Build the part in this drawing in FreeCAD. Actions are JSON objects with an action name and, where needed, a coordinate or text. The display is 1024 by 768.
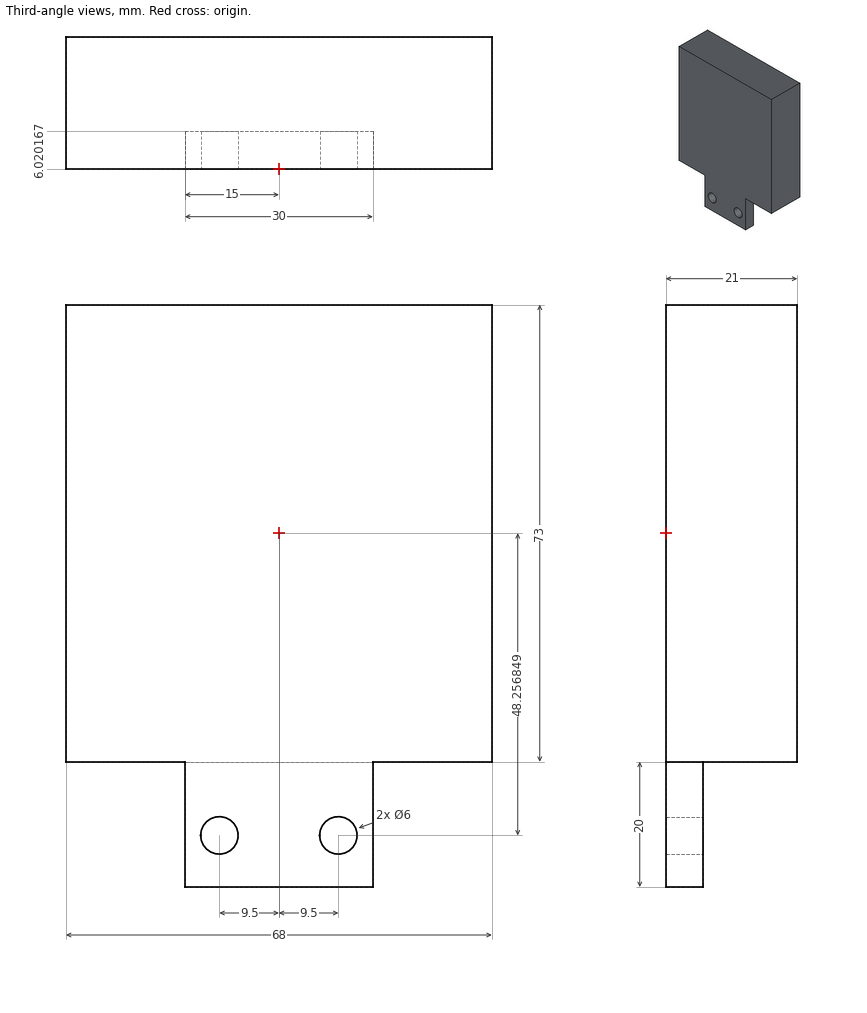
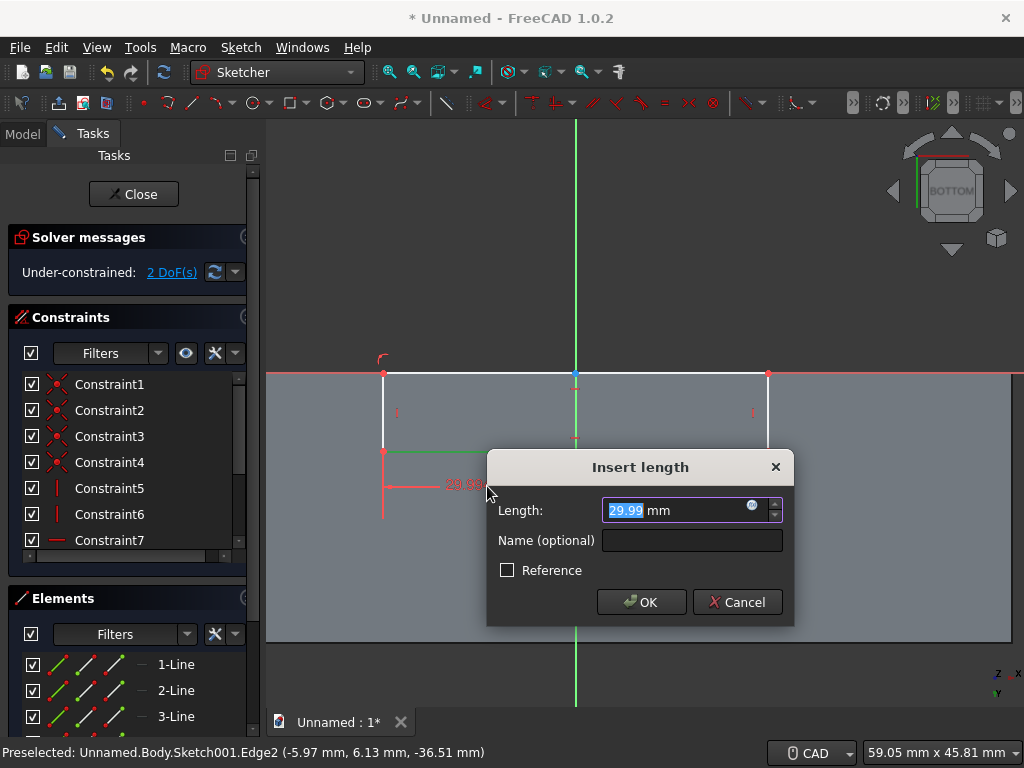
{"action": "type", "text": "30"}
{"action": "key", "text": "Return"}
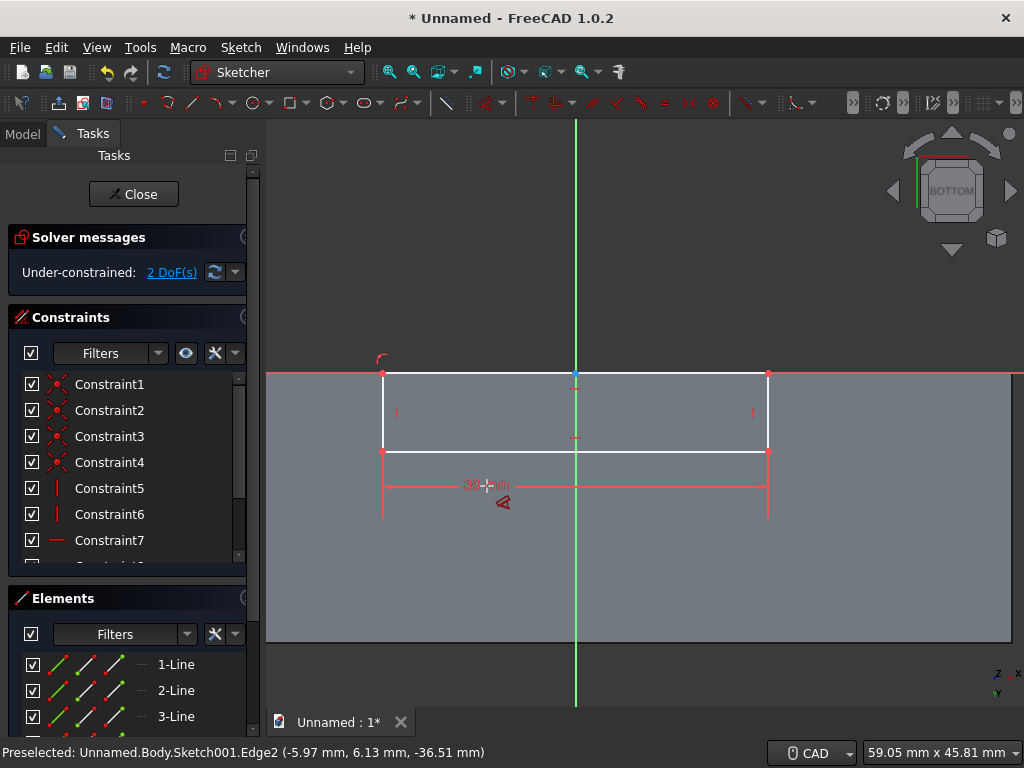
{"action": "left_click", "coordinate": [383, 373]}
{"action": "left_click", "coordinate": [479, 339]}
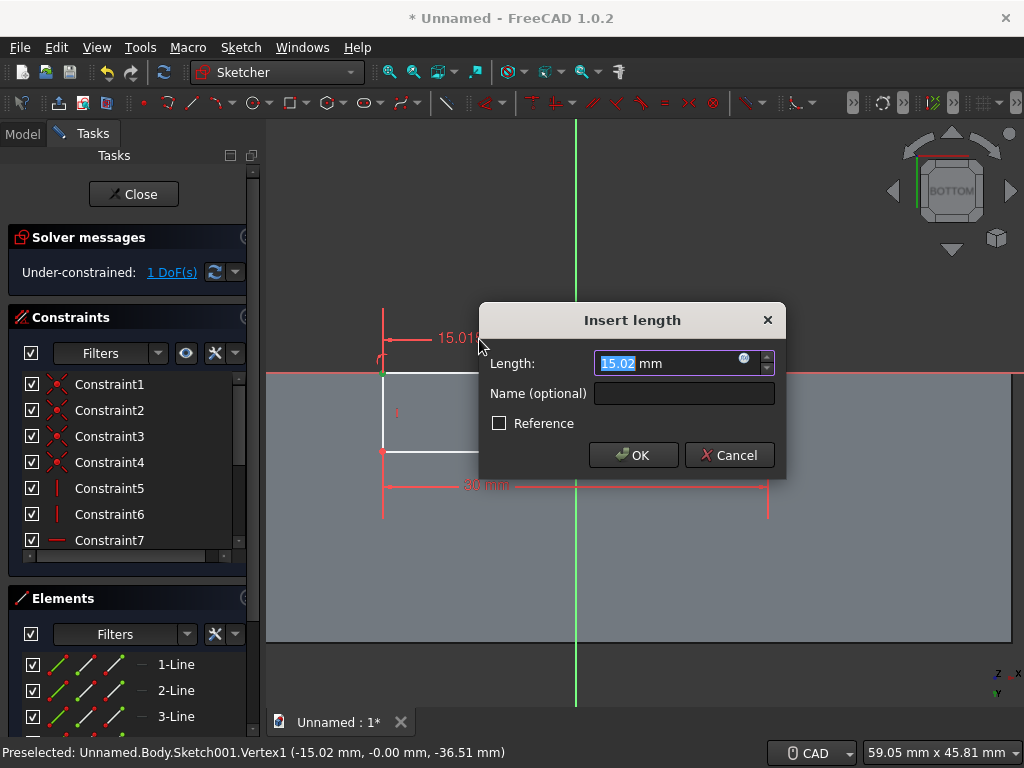
{"action": "type", "text": "15"}
{"action": "key", "text": "Return"}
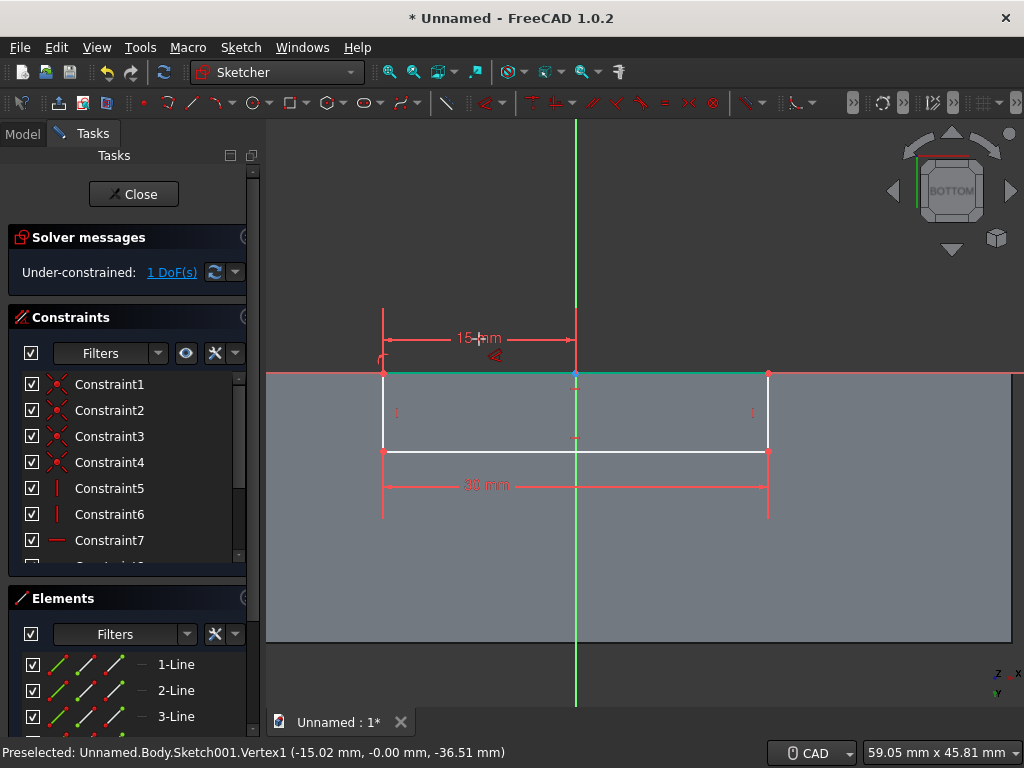
{"action": "left_click", "coordinate": [383, 397]}
{"action": "left_click", "coordinate": [349, 413]}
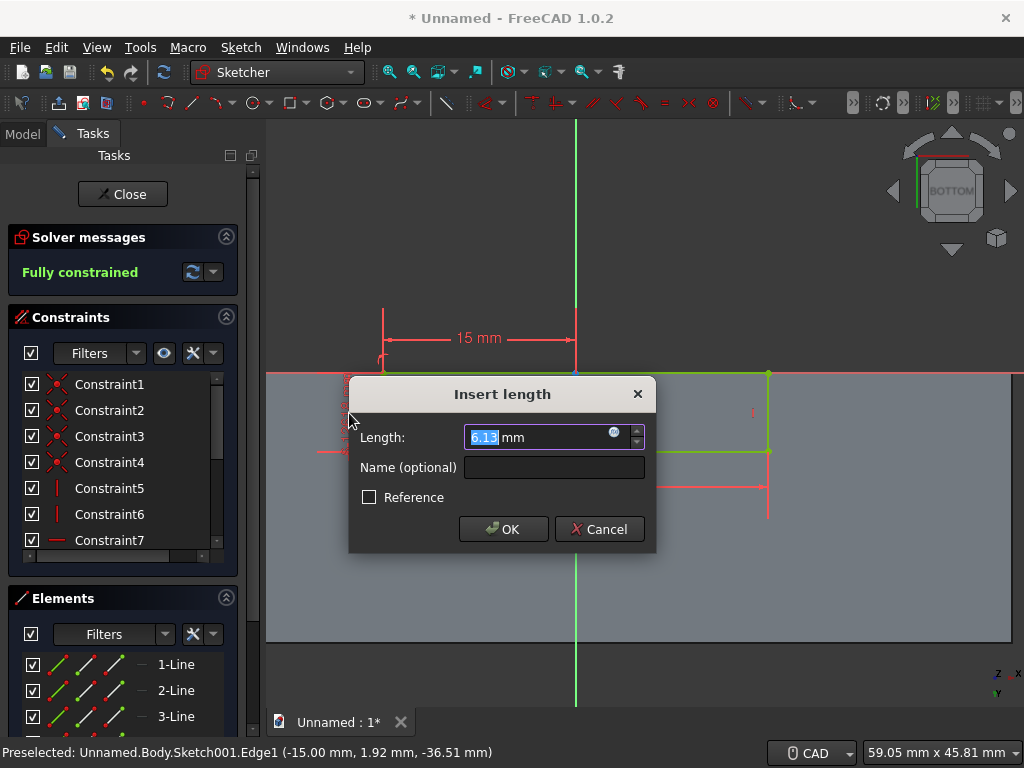
{"action": "type", "text": "6.020167"}
{"action": "key", "text": "Return"}
{"action": "key", "text": "Escape"}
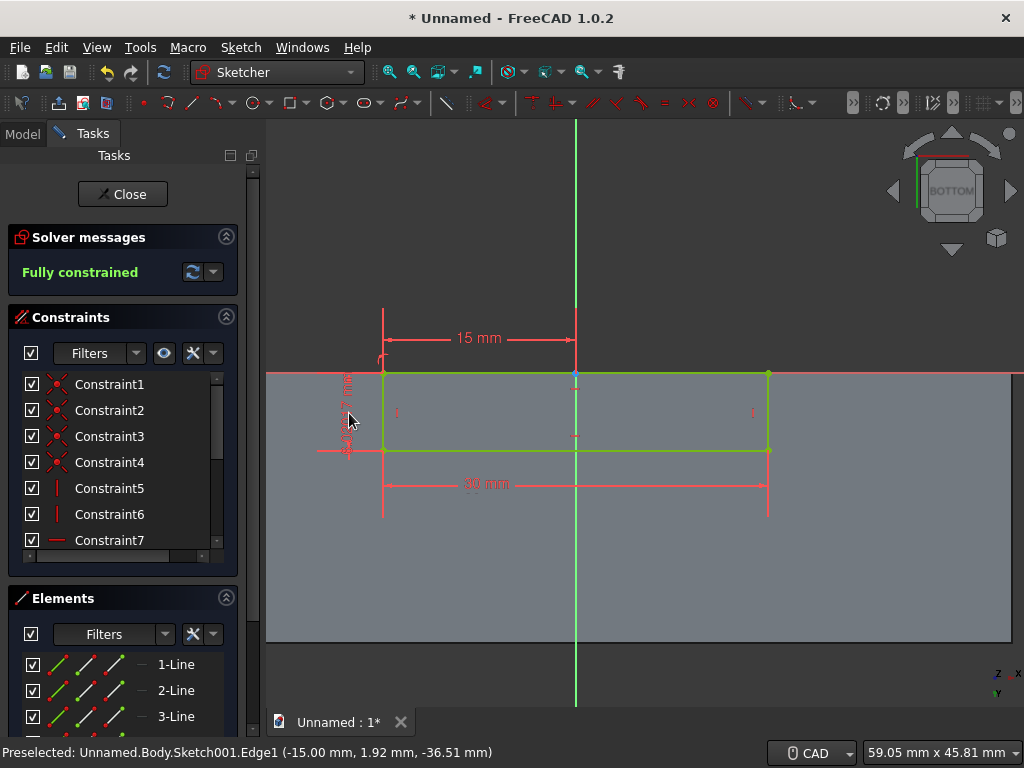
{"action": "left_click", "coordinate": [123, 194]}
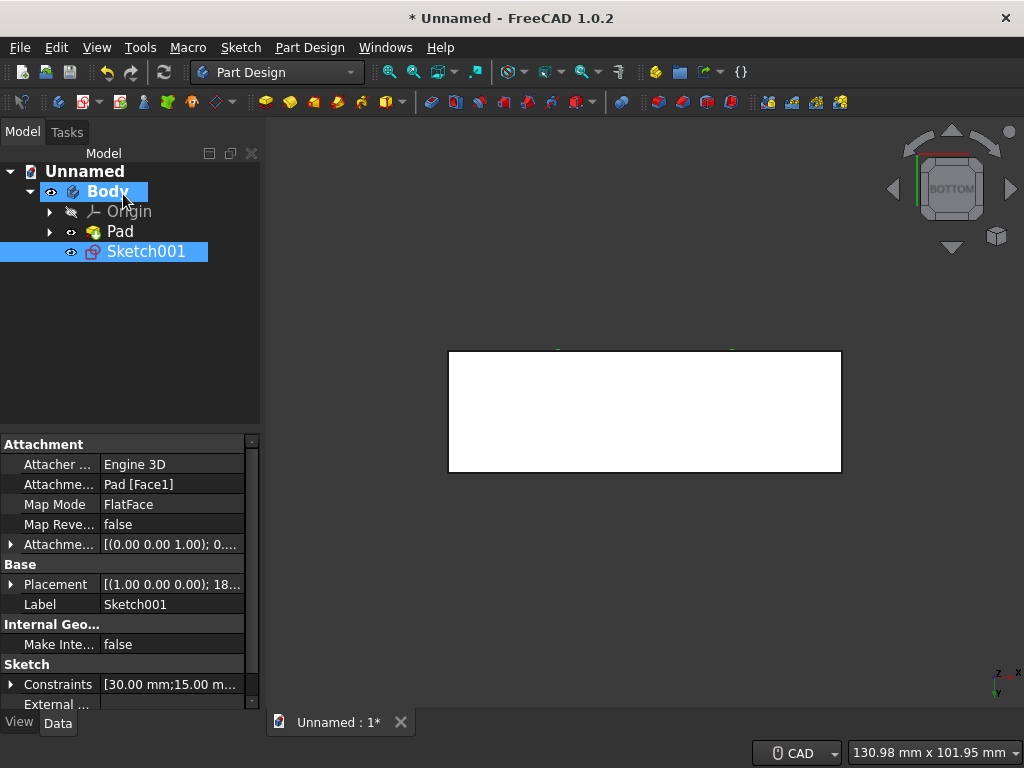
{"action": "left_click", "coordinate": [266, 102]}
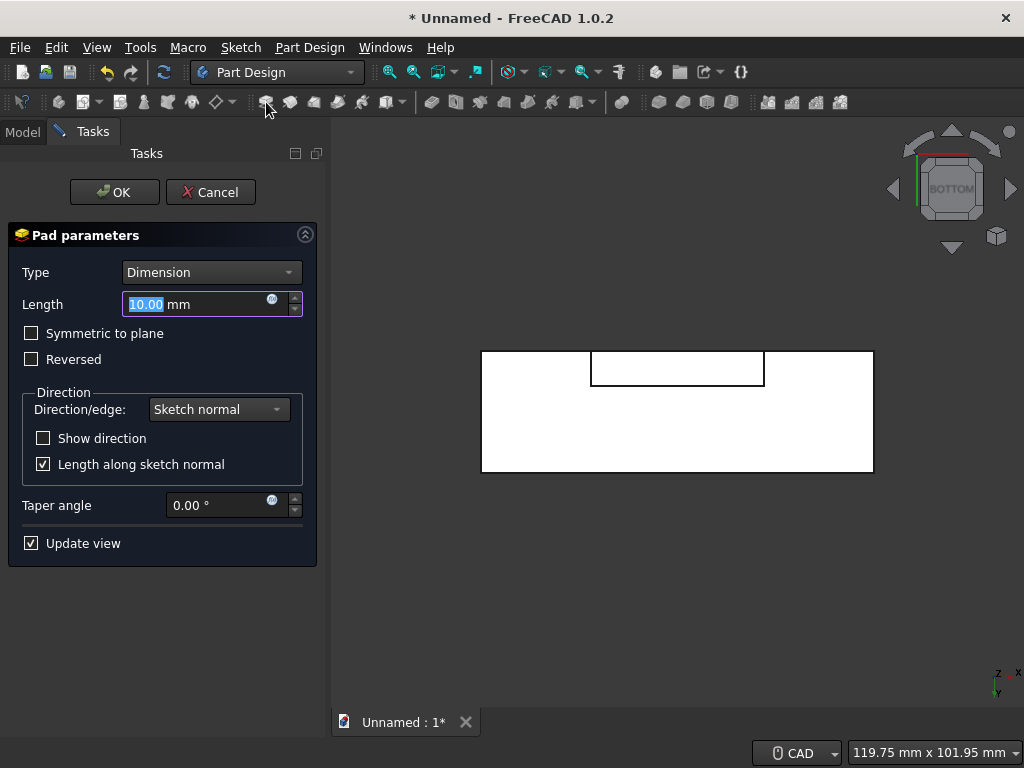
{"action": "type", "text": "20"}
{"action": "key", "text": "Tab"}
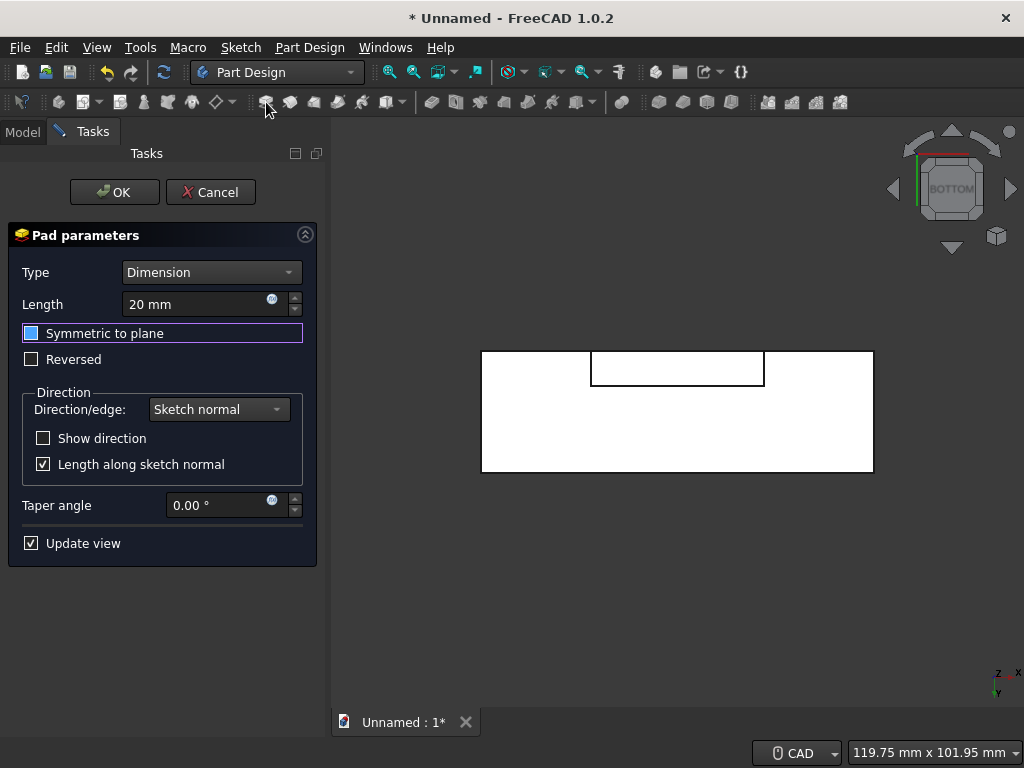
{"action": "left_click", "coordinate": [115, 192]}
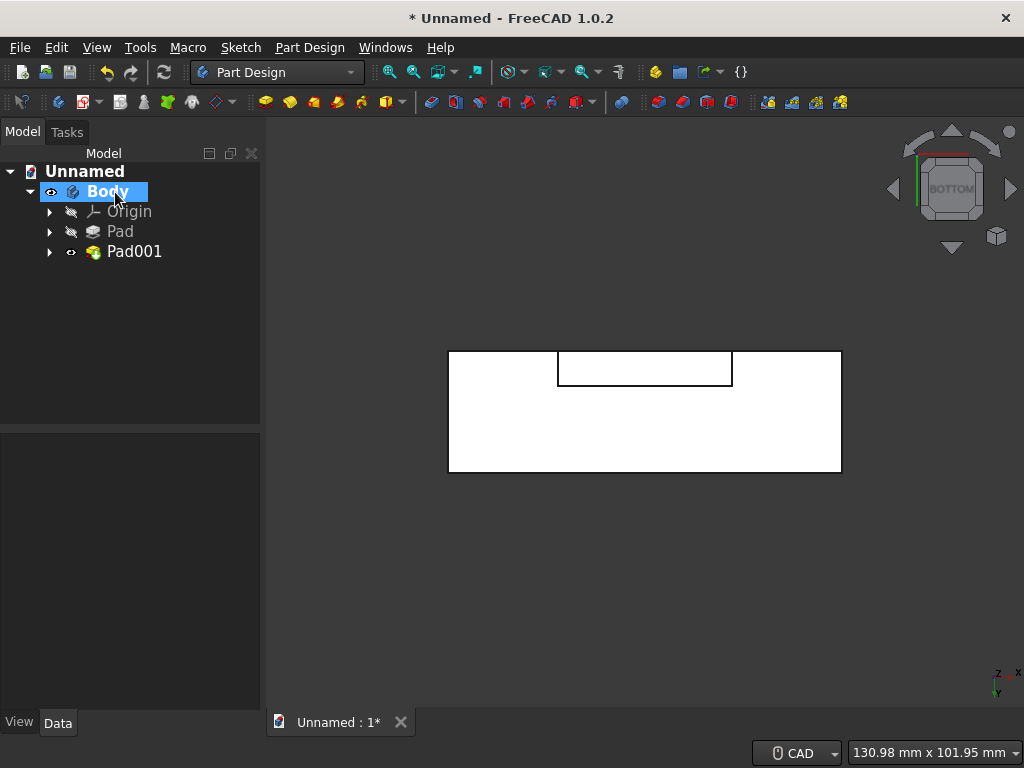
{"action": "key", "text": "4"}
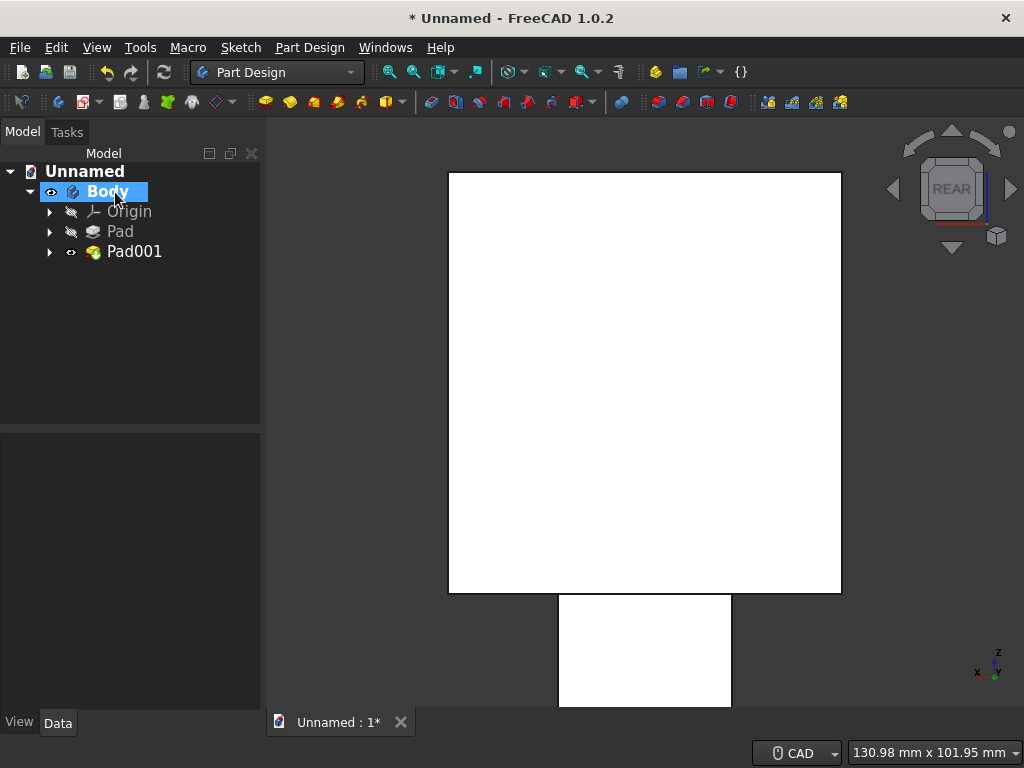
{"action": "key", "text": "v f"}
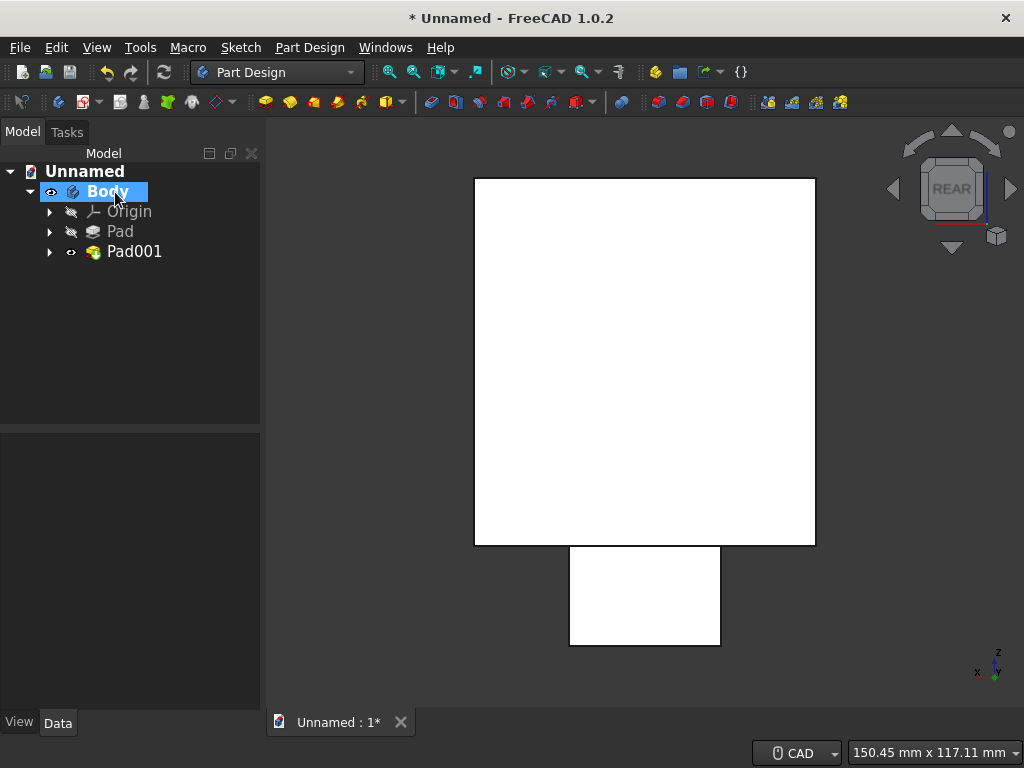
{"action": "left_click", "coordinate": [623, 595]}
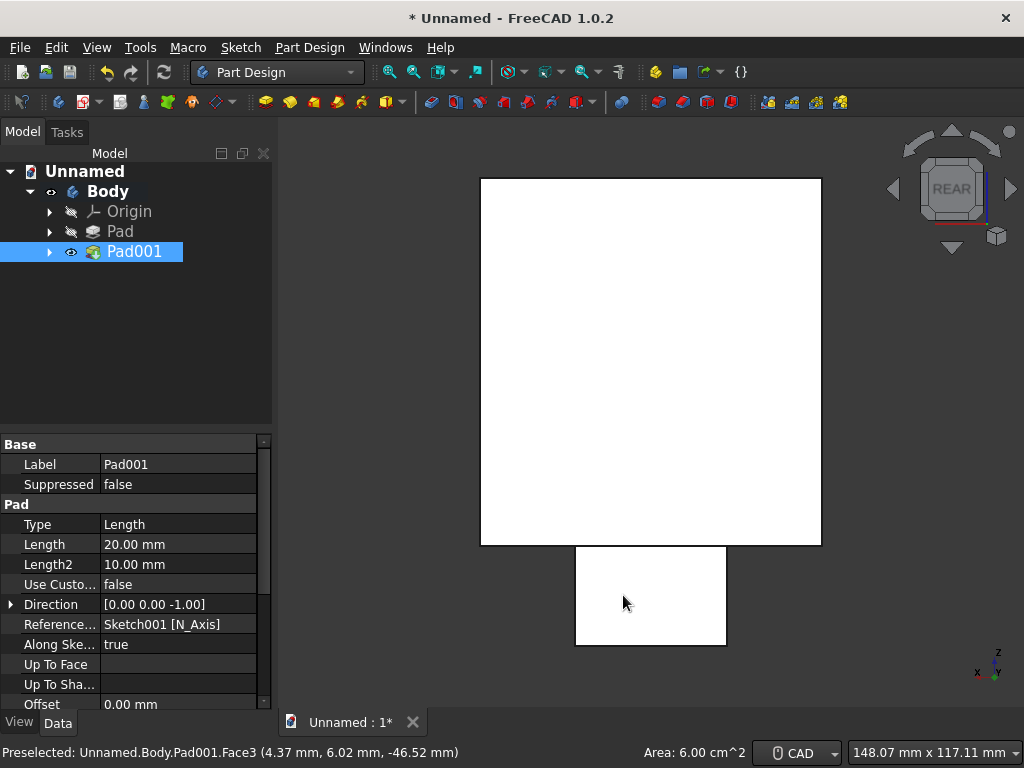
{"action": "left_click", "coordinate": [84, 102]}